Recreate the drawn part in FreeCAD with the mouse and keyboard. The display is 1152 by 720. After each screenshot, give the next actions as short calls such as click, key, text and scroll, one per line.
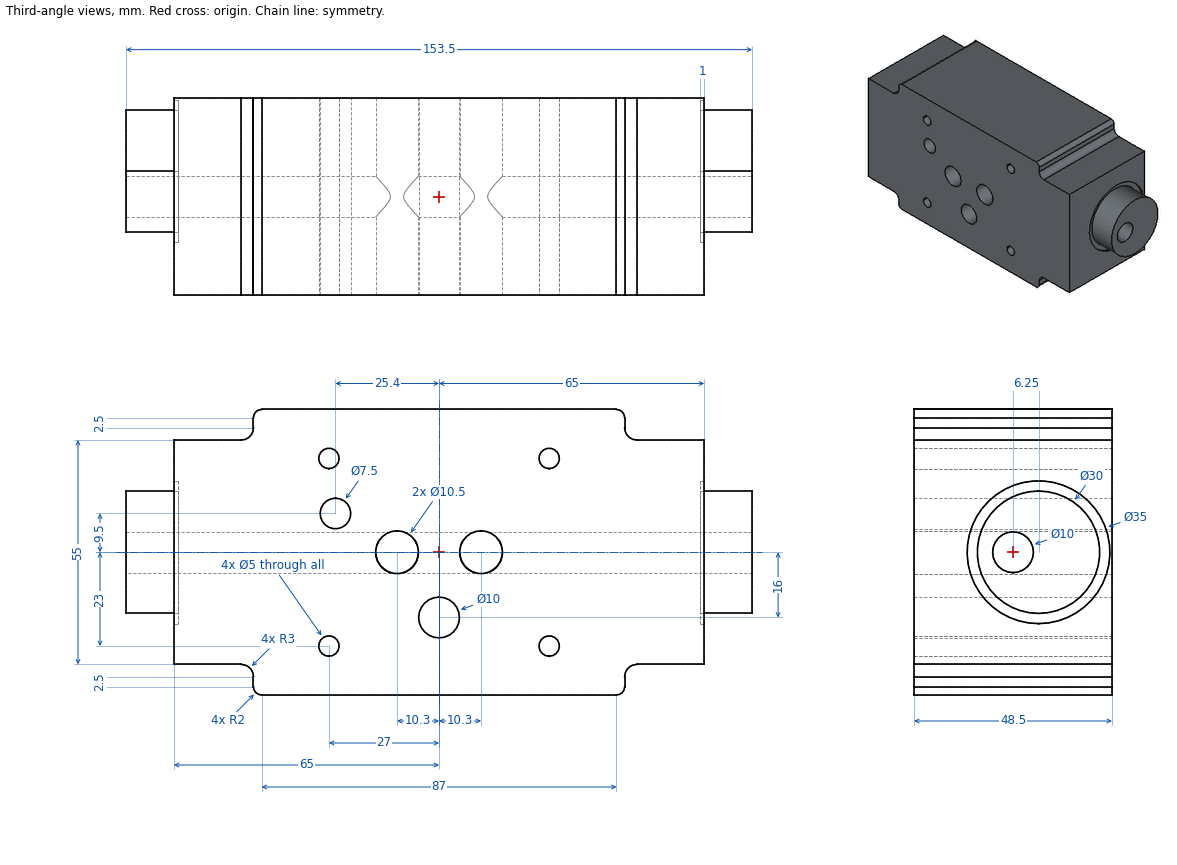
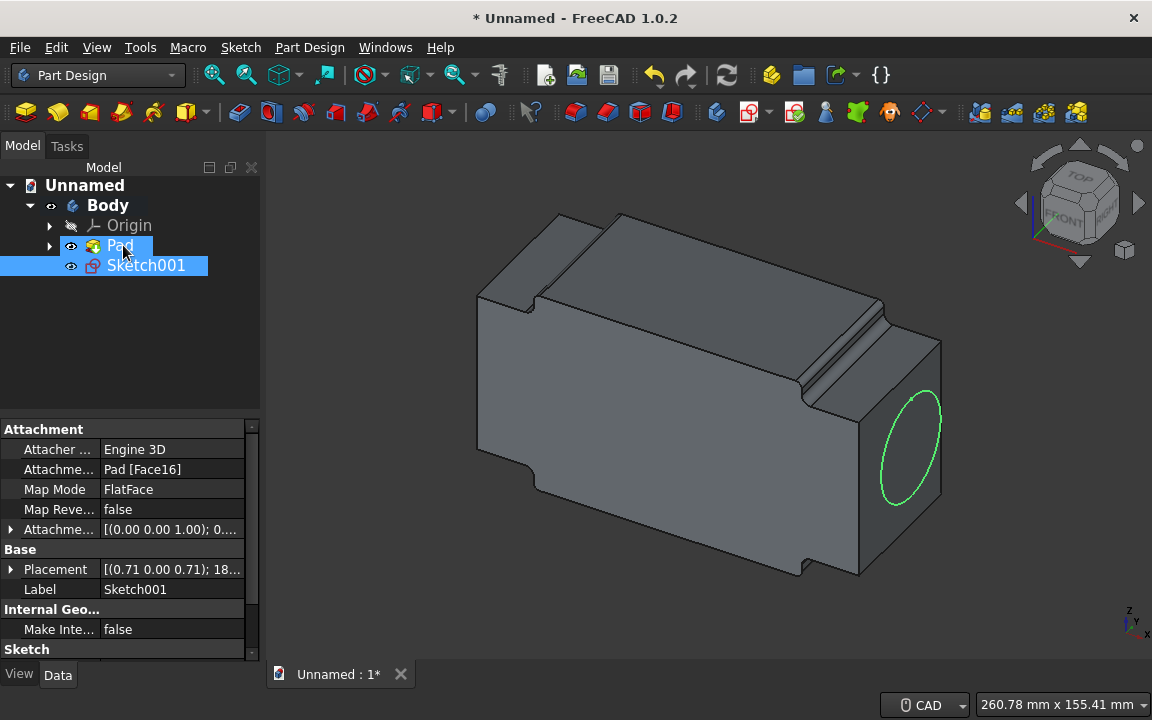
click(240, 112)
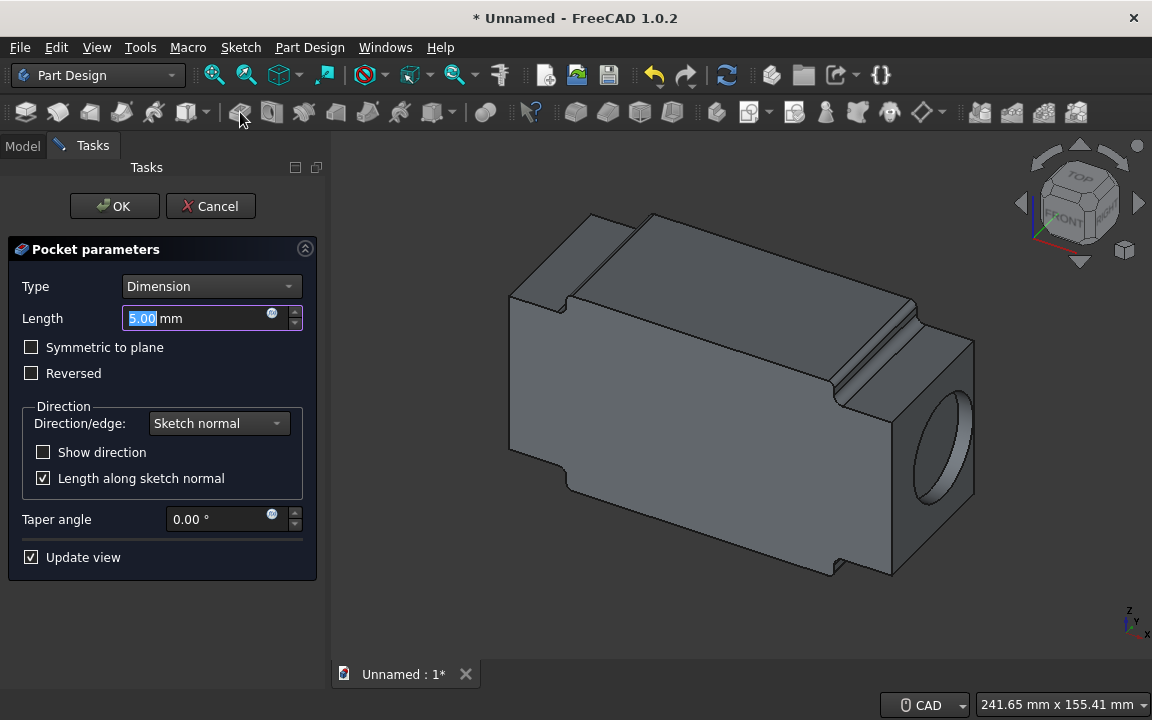
text(1)
key(Tab)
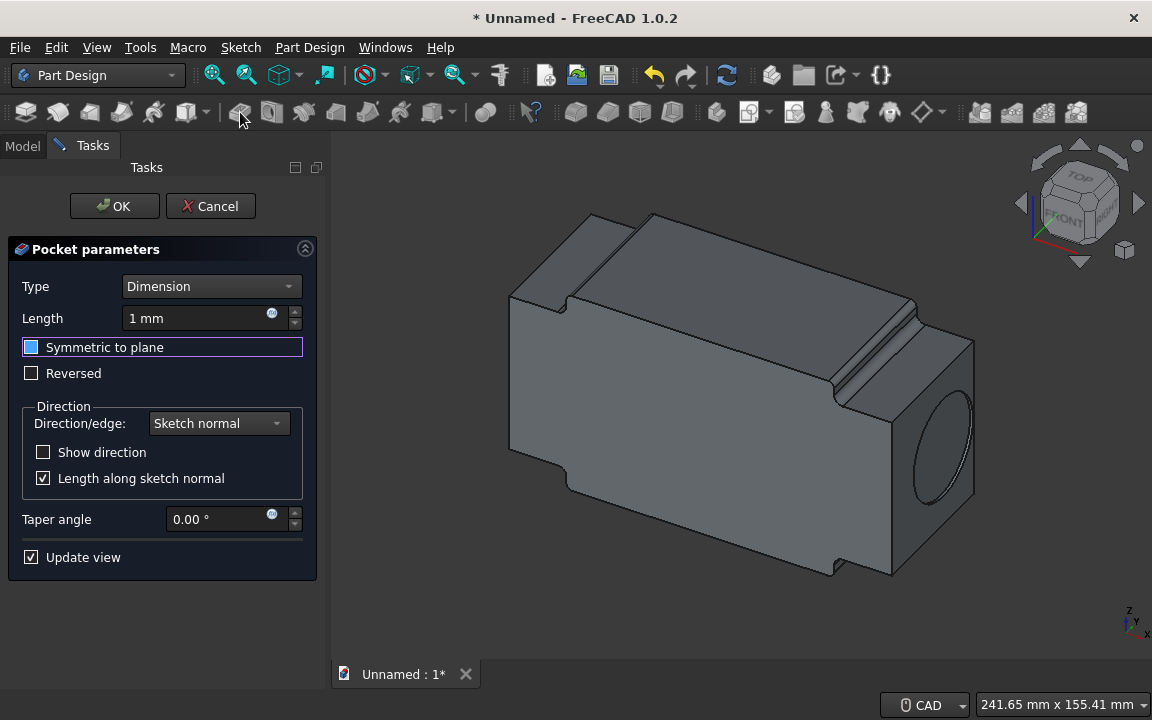
click(115, 206)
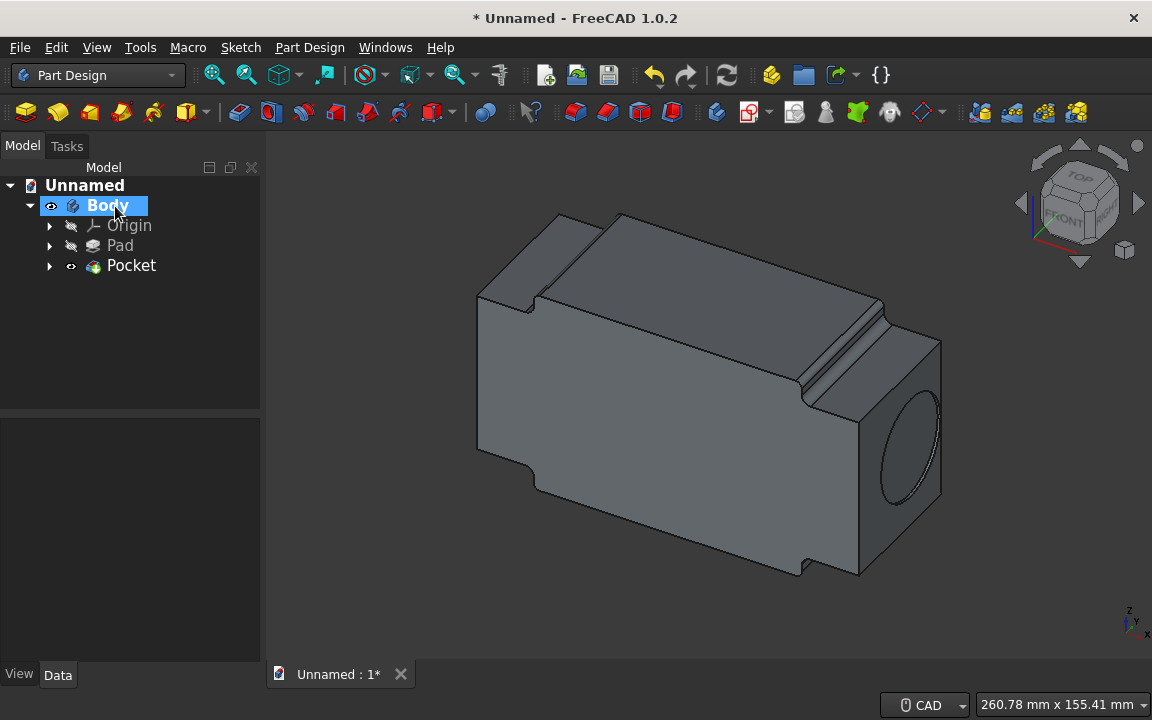
click(116, 266)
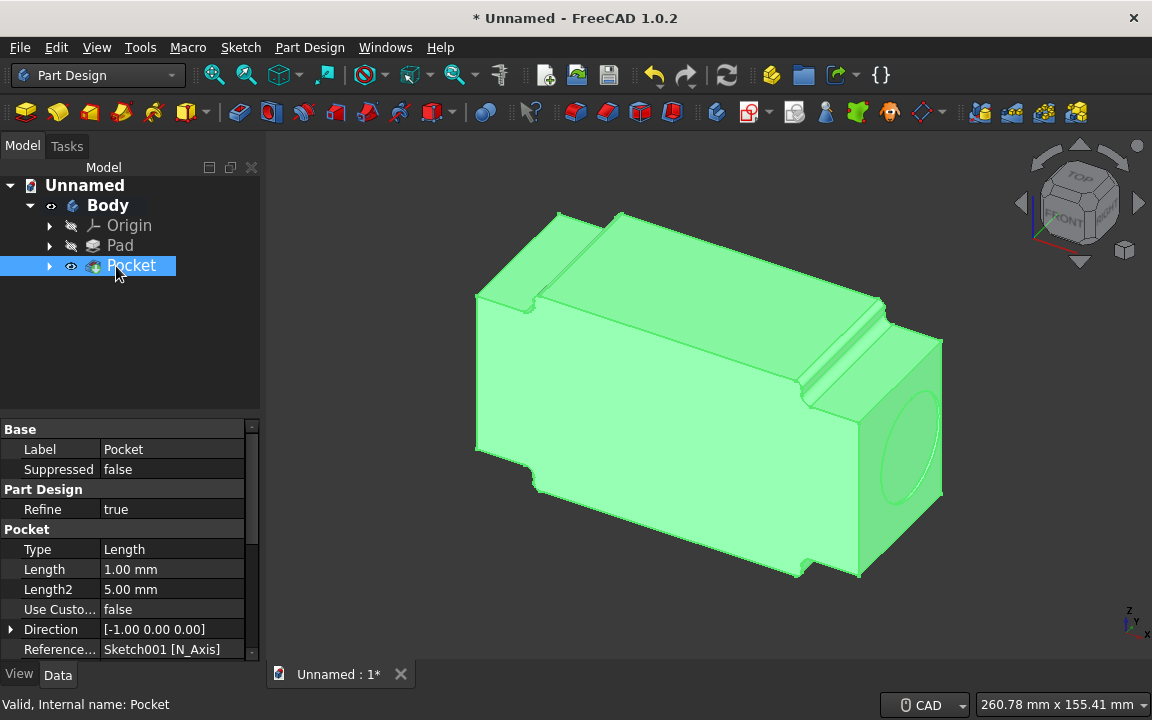
click(980, 112)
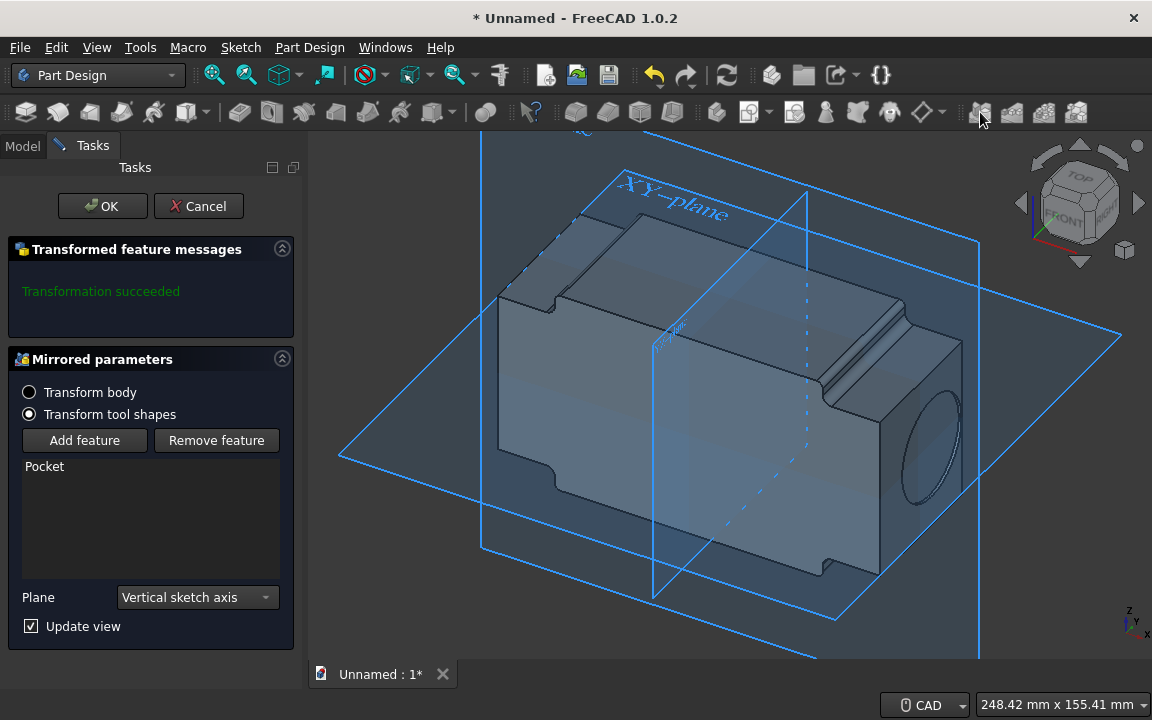
click(198, 598)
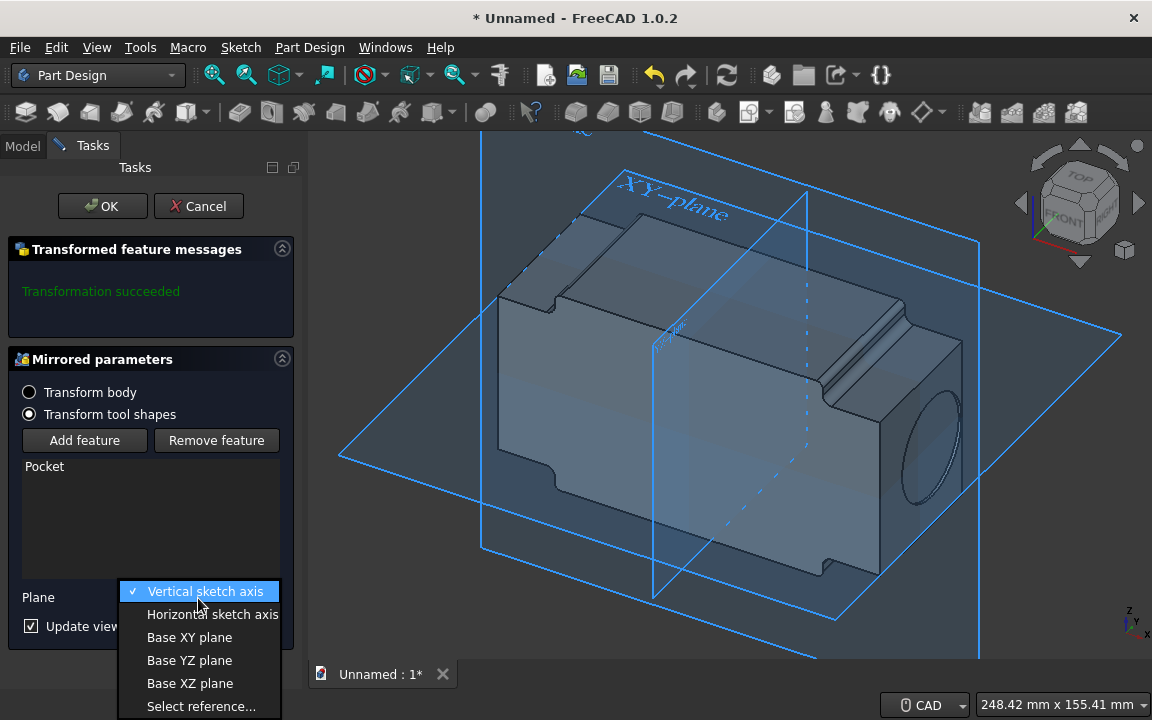
click(198, 660)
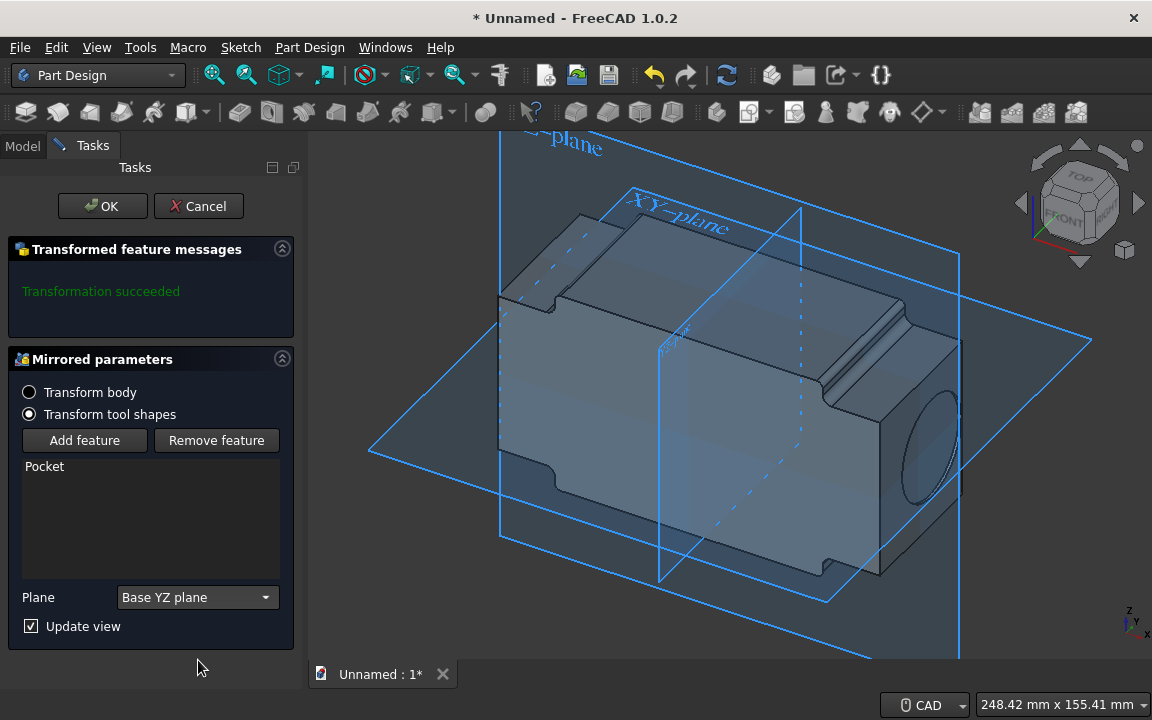
click(103, 206)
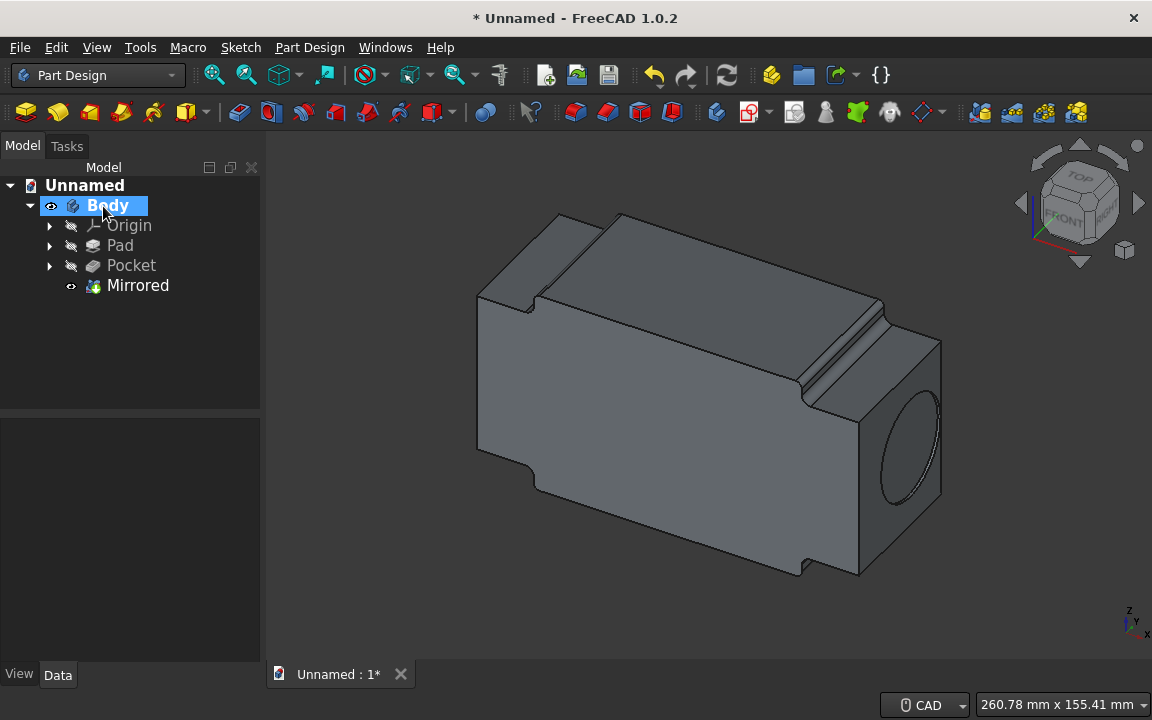
click(750, 112)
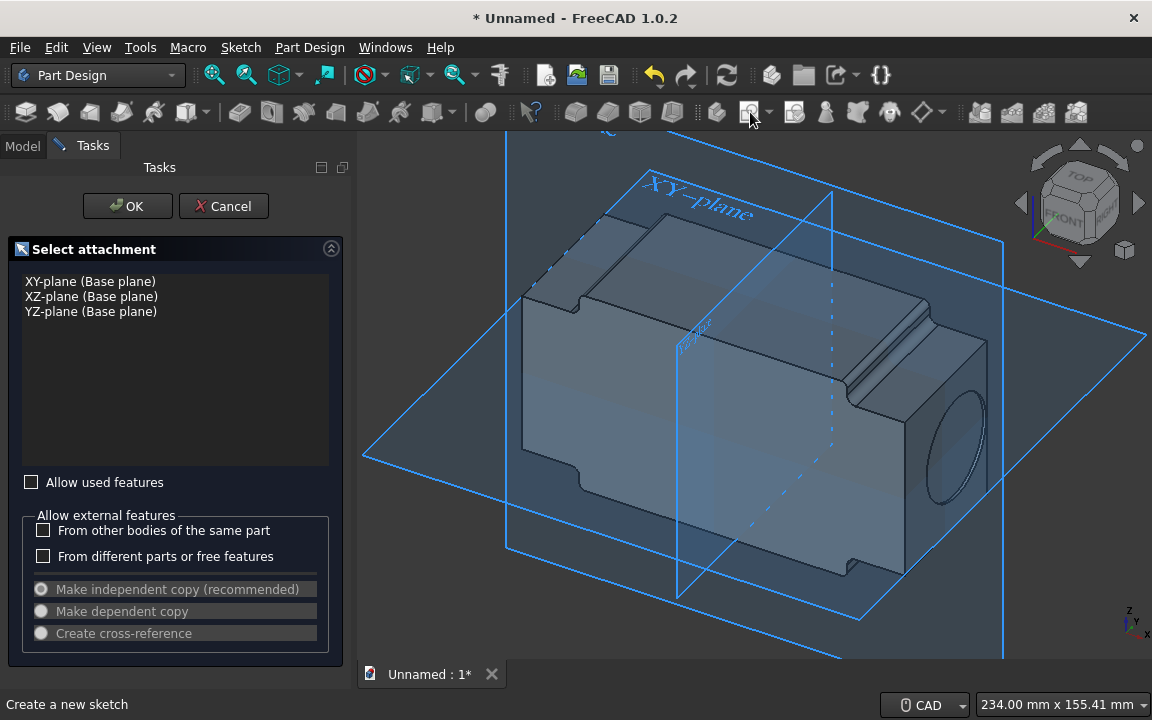
click(82, 312)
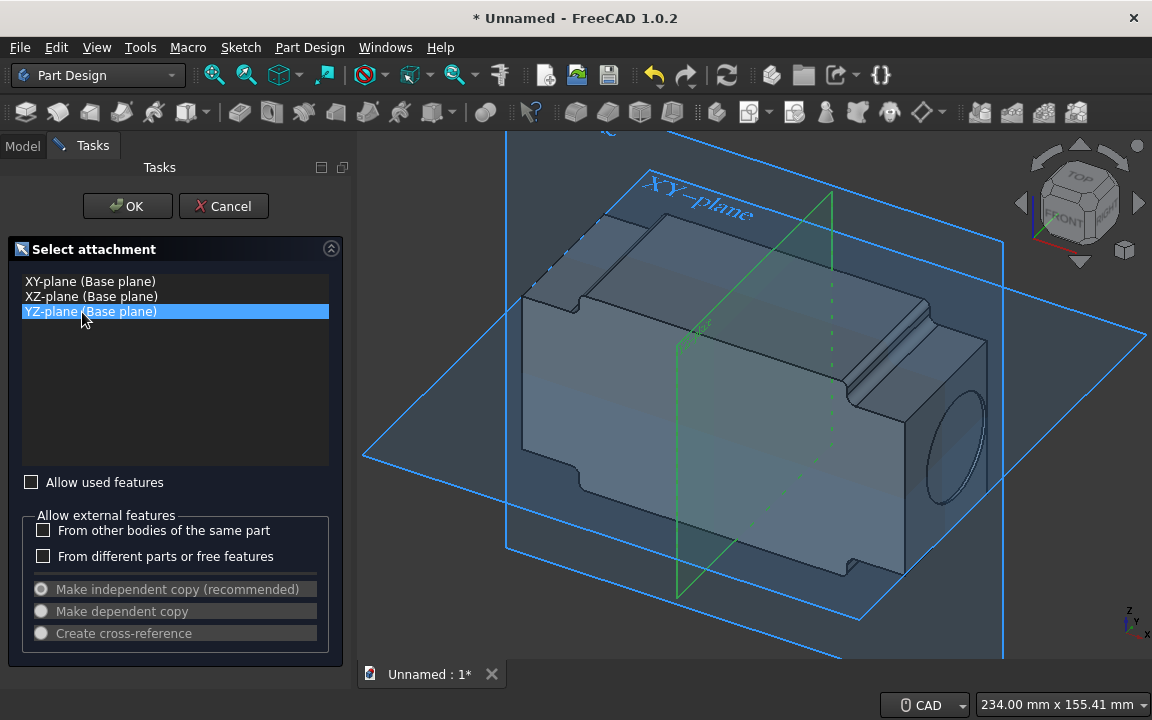
click(128, 206)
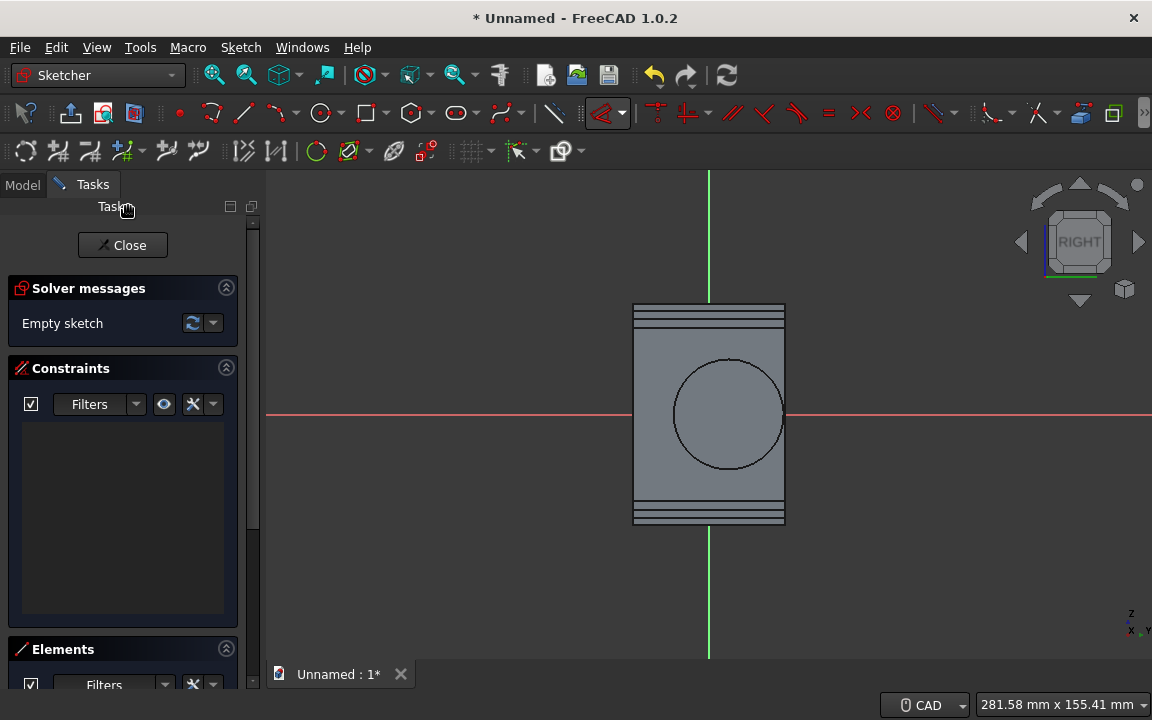
click(136, 114)